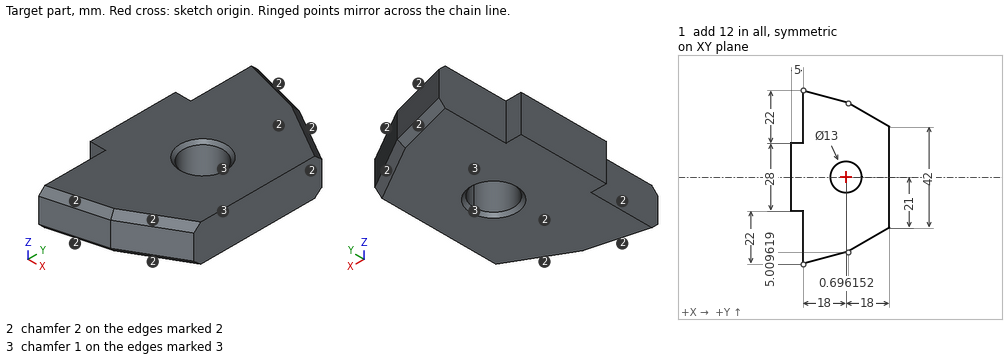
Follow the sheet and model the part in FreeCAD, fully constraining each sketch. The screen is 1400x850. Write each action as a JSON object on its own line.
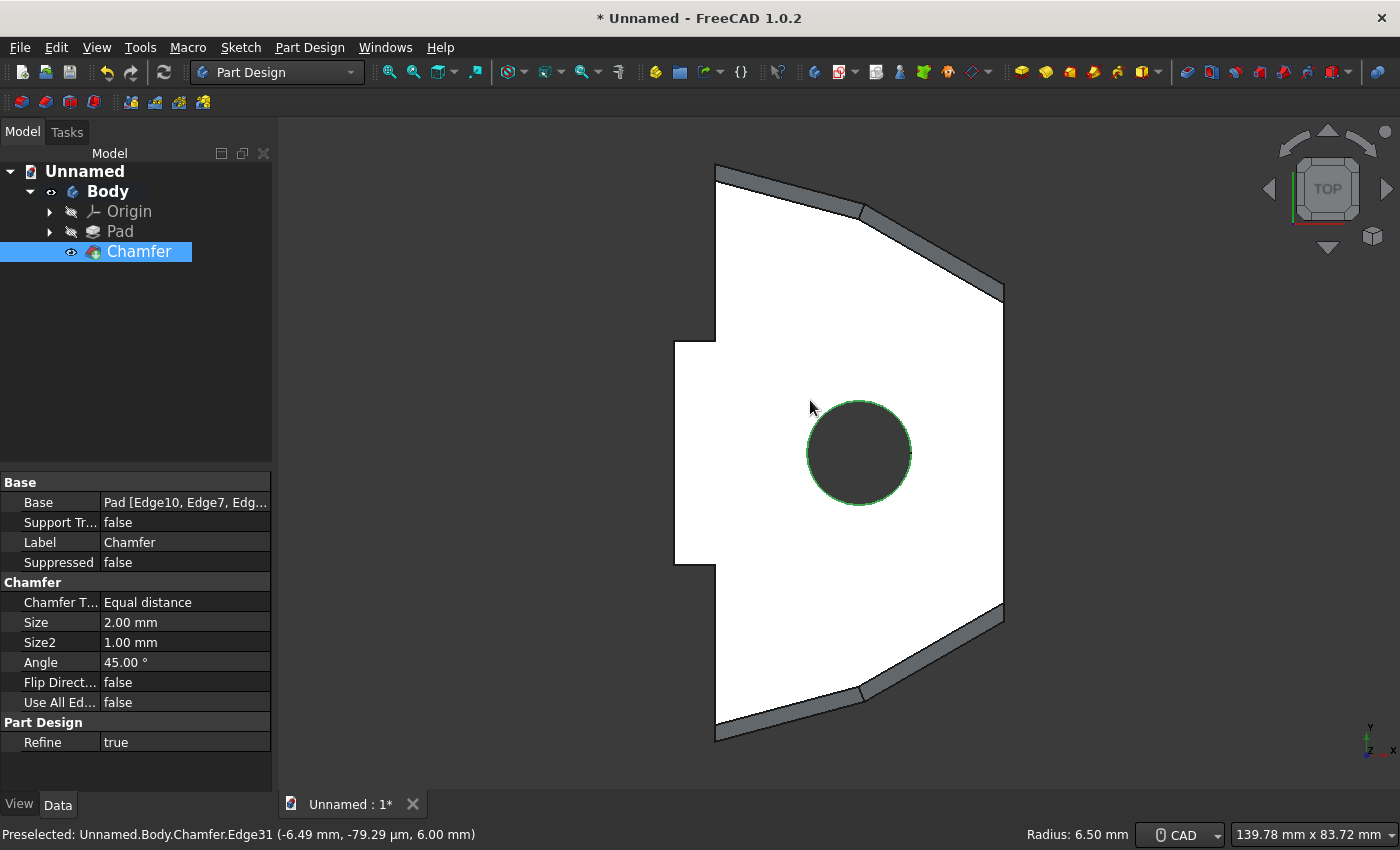
{"action": "key", "text": "1"}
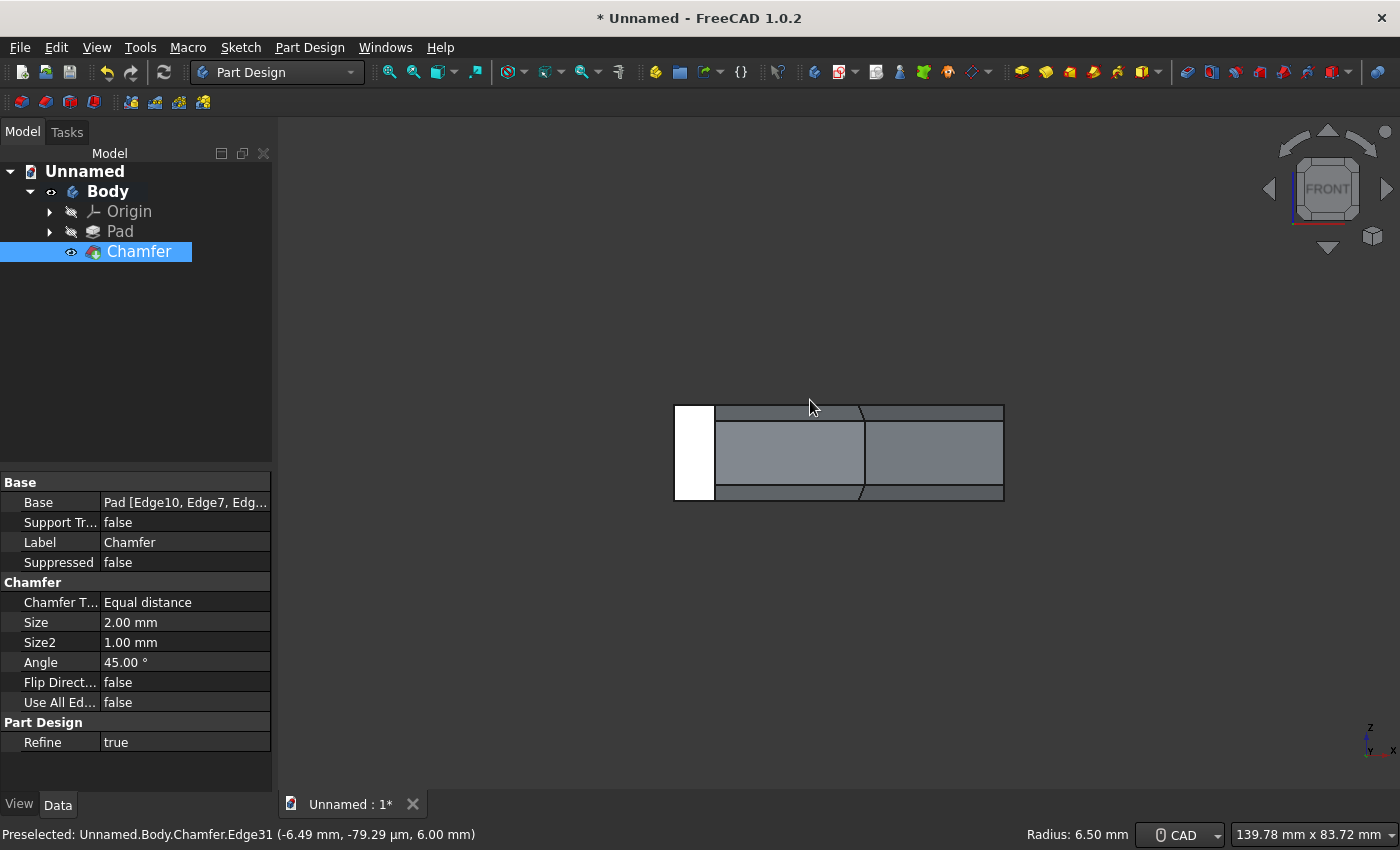
{"action": "left_click", "coordinate": [390, 72]}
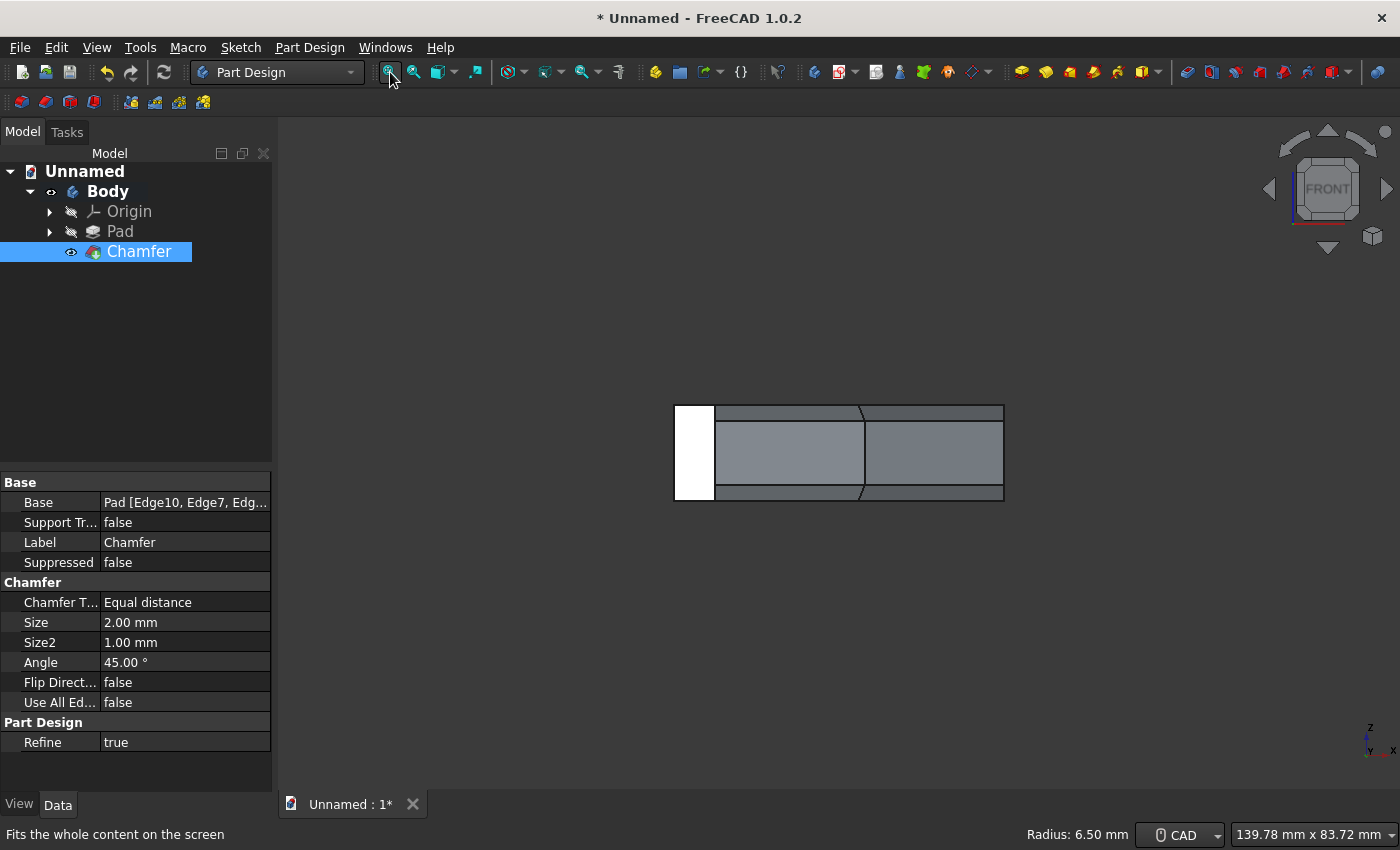
{"action": "key", "text": "3"}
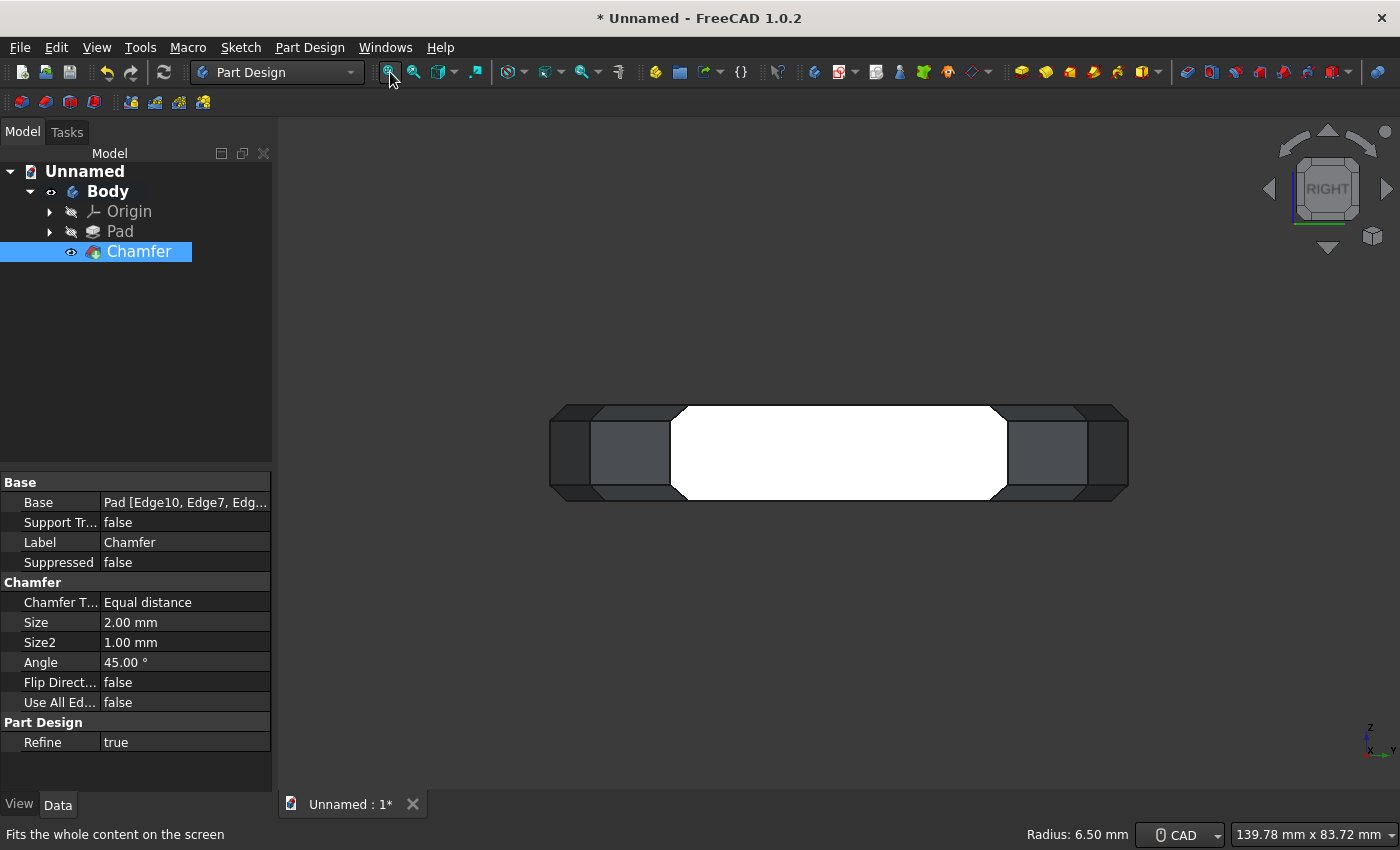
{"action": "key", "text": "5"}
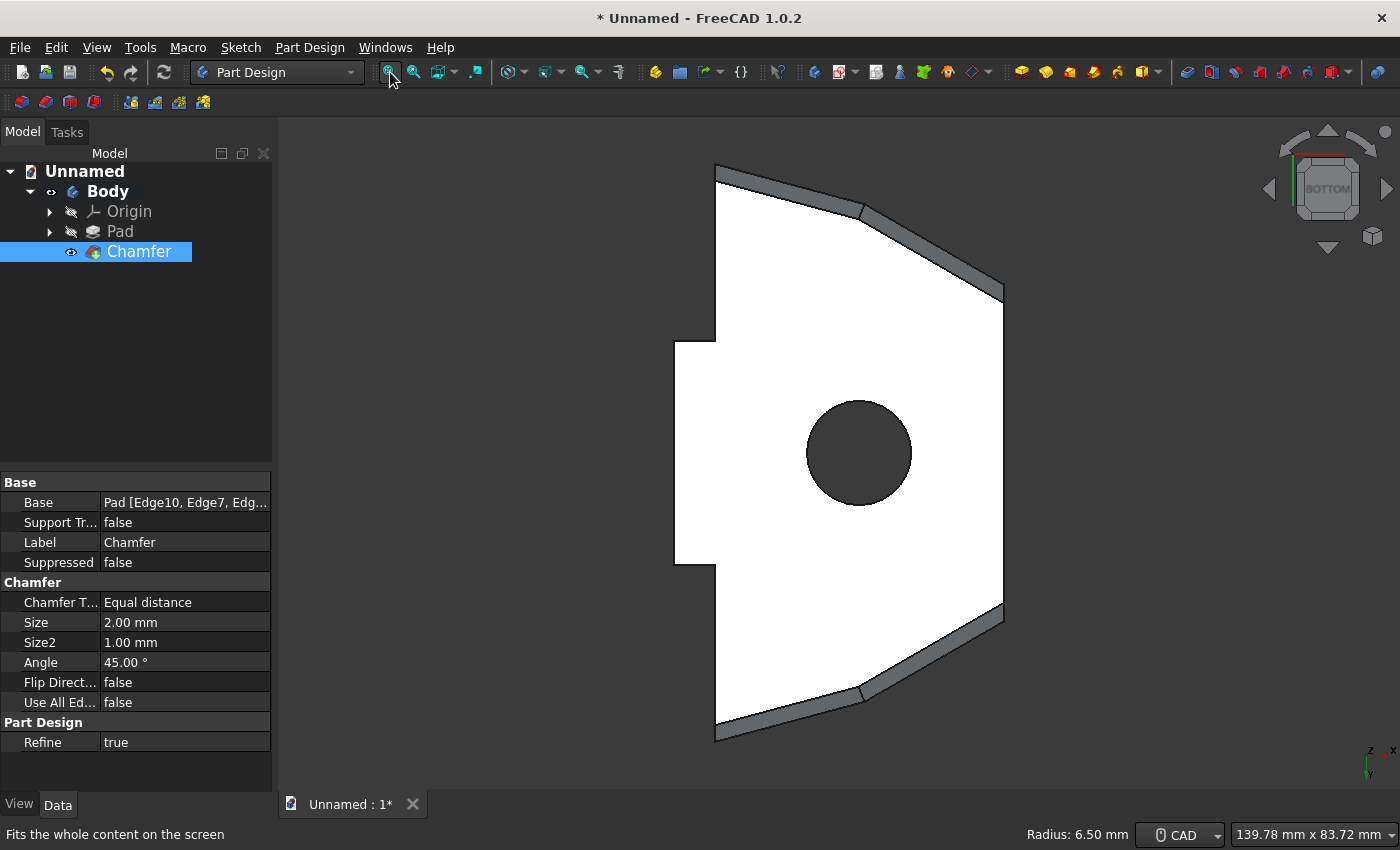
{"action": "left_click", "coordinate": [807, 452], "text": "ctrl"}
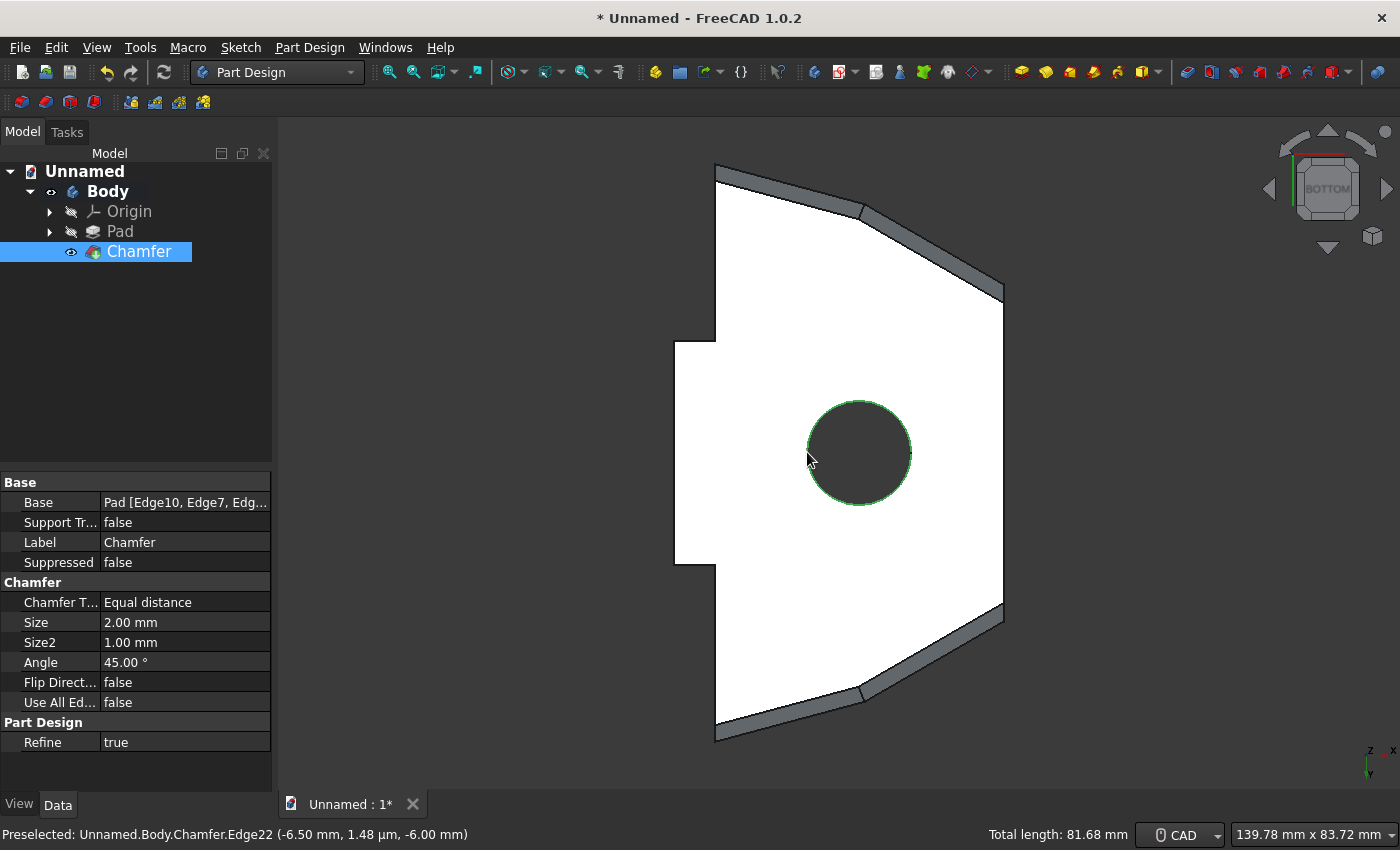
{"action": "left_click", "coordinate": [46, 102]}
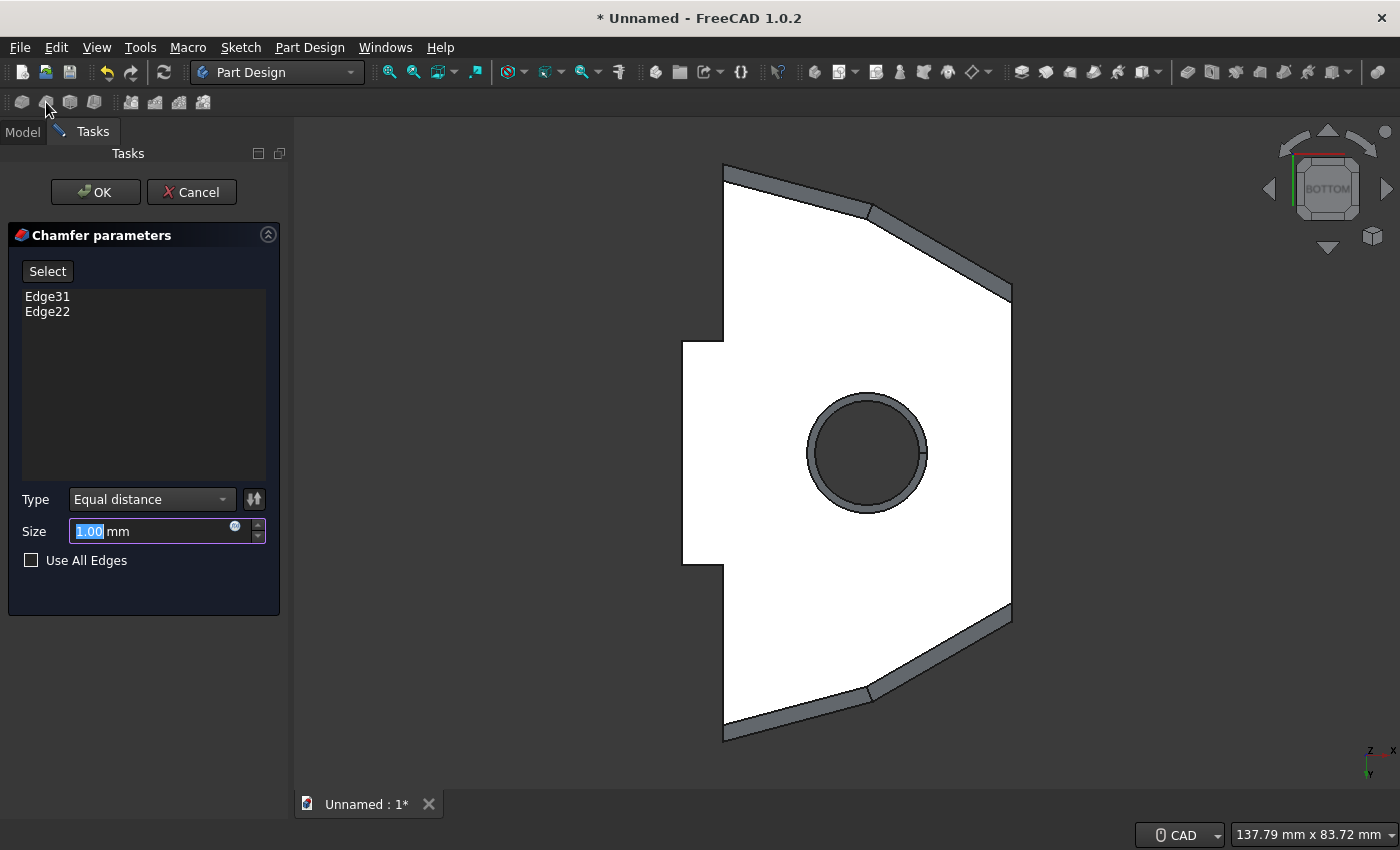
{"action": "type", "text": "1"}
{"action": "key", "text": "Tab"}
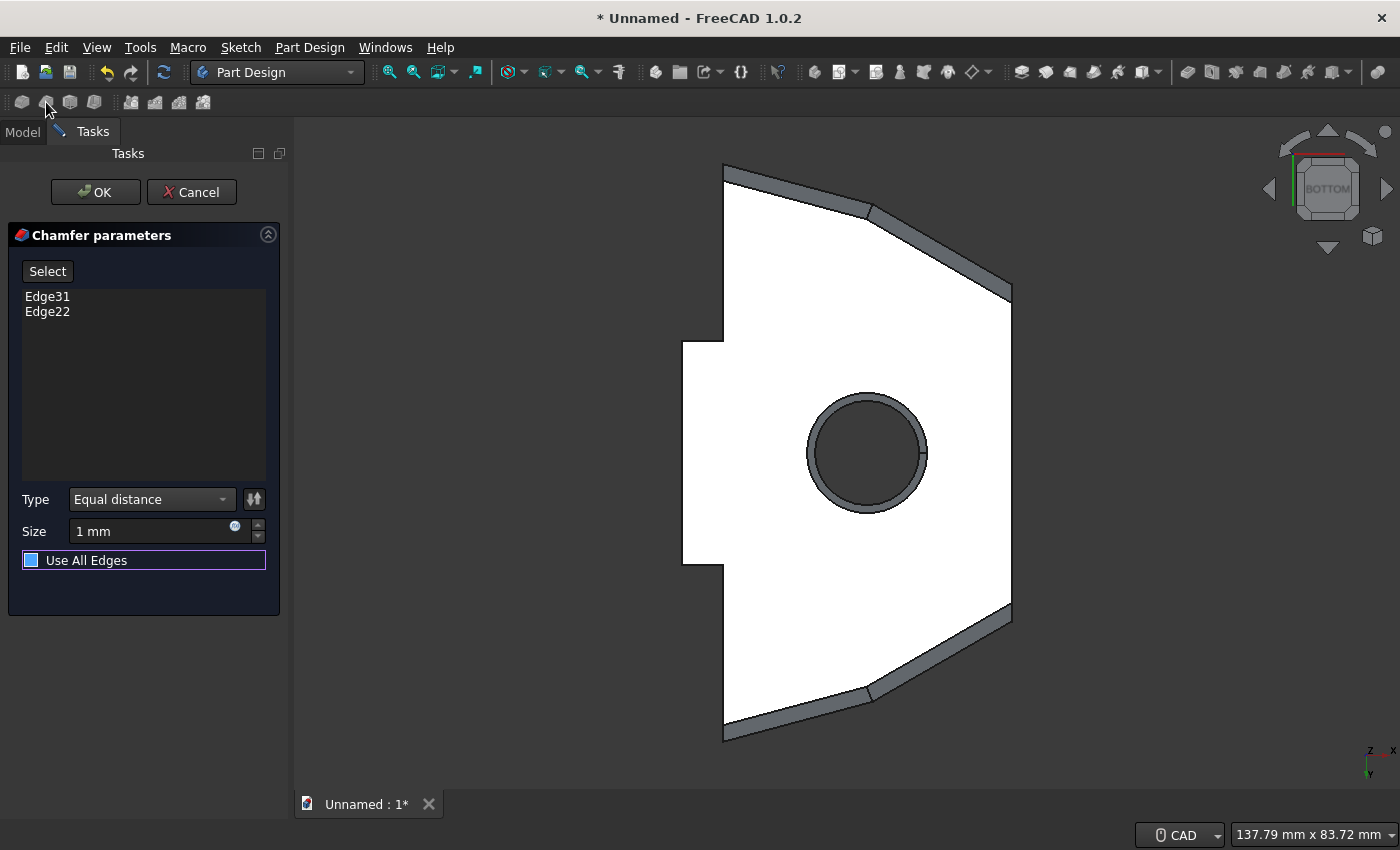
{"action": "left_click", "coordinate": [96, 192]}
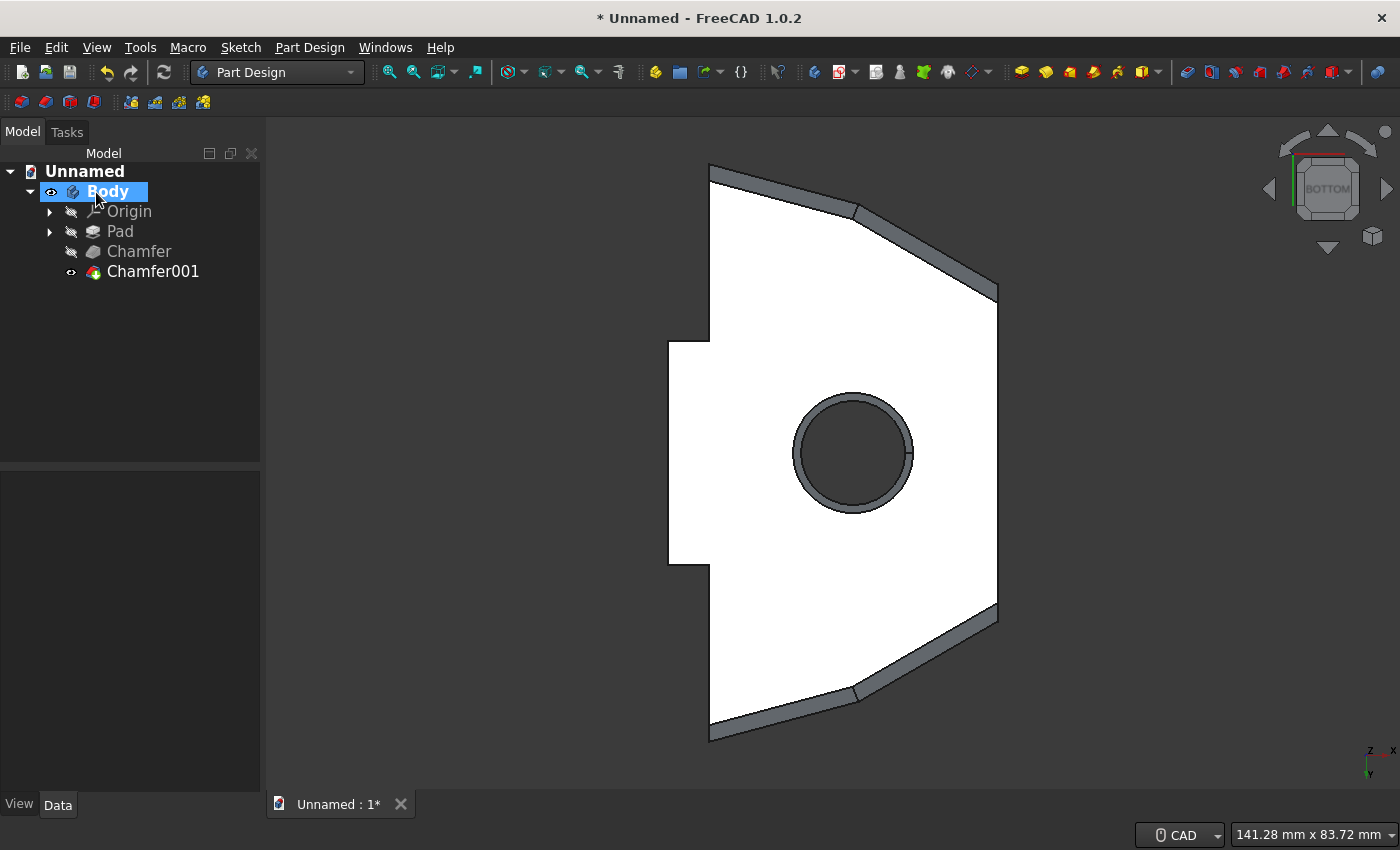
{"action": "key", "text": "0"}